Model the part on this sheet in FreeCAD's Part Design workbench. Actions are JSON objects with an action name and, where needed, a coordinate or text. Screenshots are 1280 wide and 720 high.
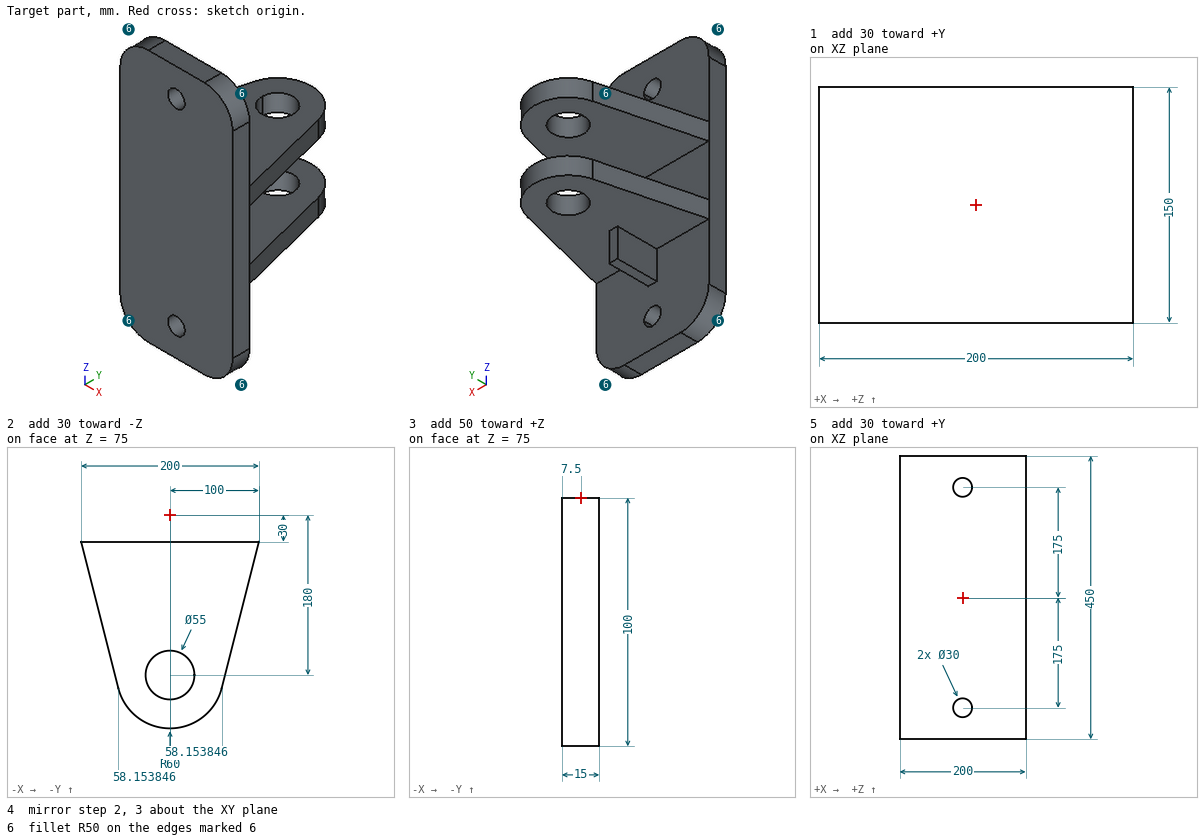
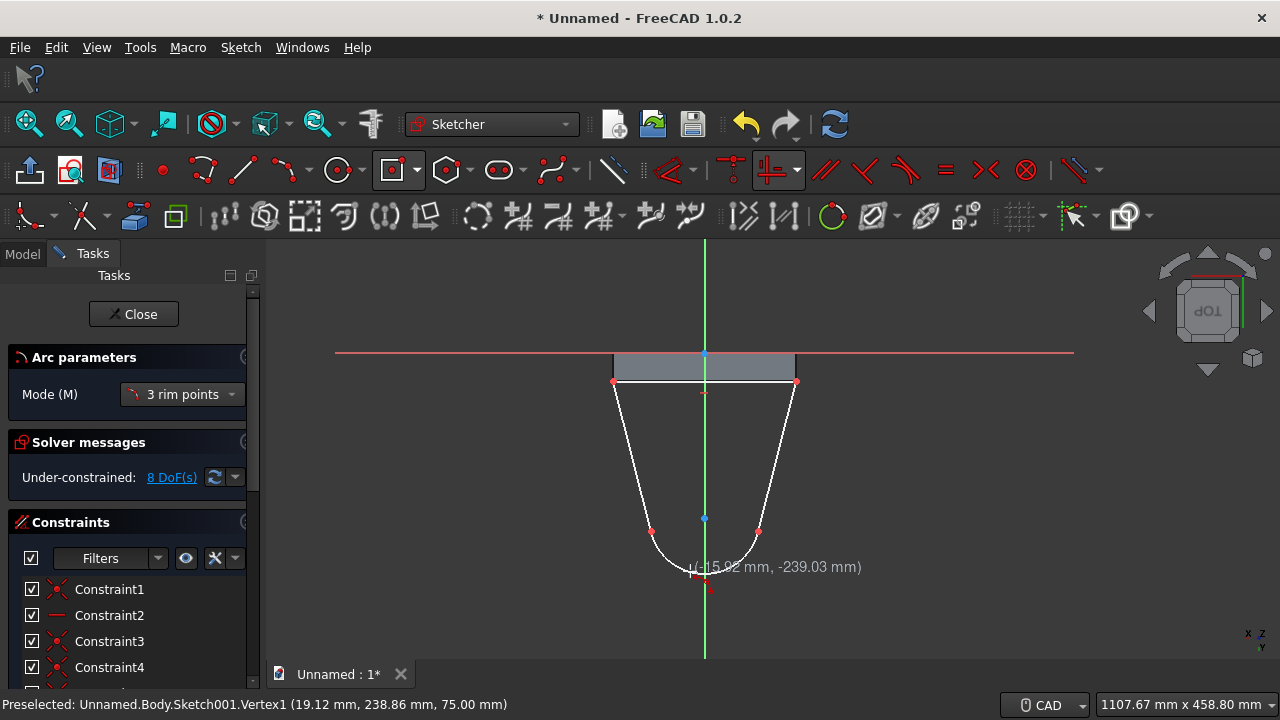
{"action": "key", "text": "g c"}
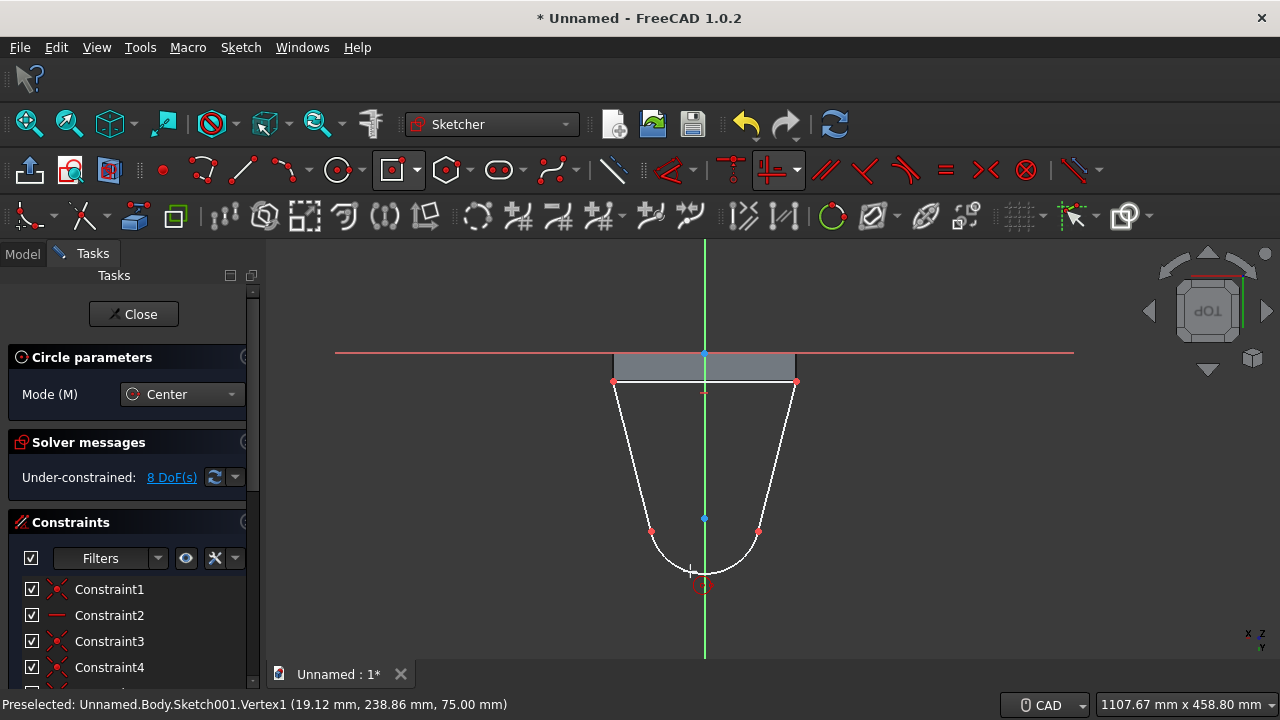
{"action": "left_click", "coordinate": [705, 518]}
{"action": "mouse_move", "coordinate": [722, 500]}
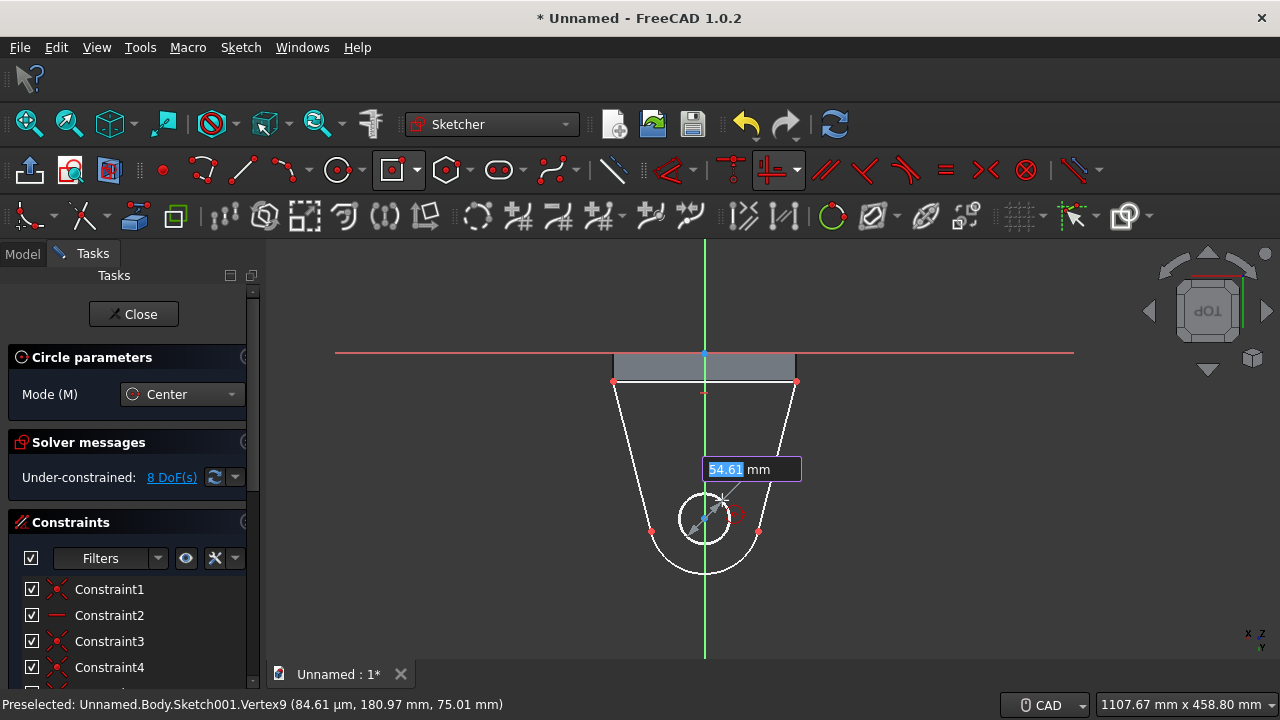
{"action": "type", "text": "55"}
{"action": "key", "text": "Return"}
{"action": "key", "text": "Escape"}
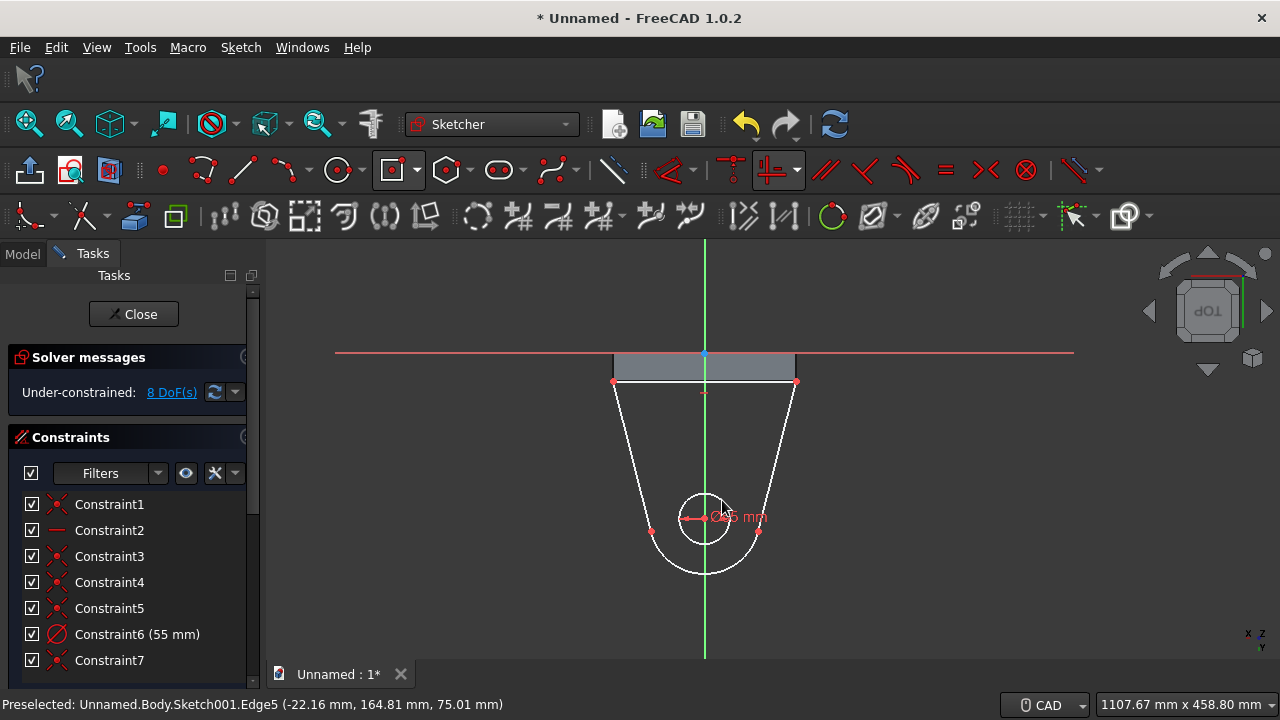
{"action": "left_click", "coordinate": [705, 519]}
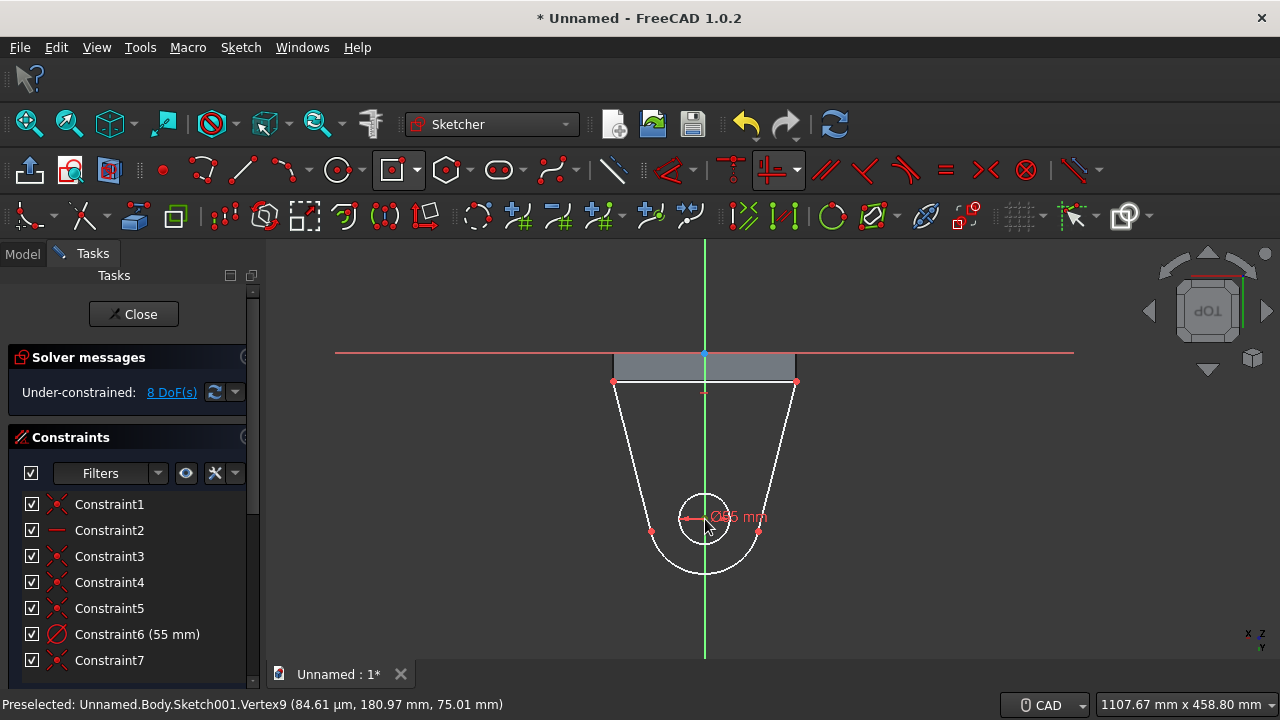
{"action": "left_click", "coordinate": [705, 605]}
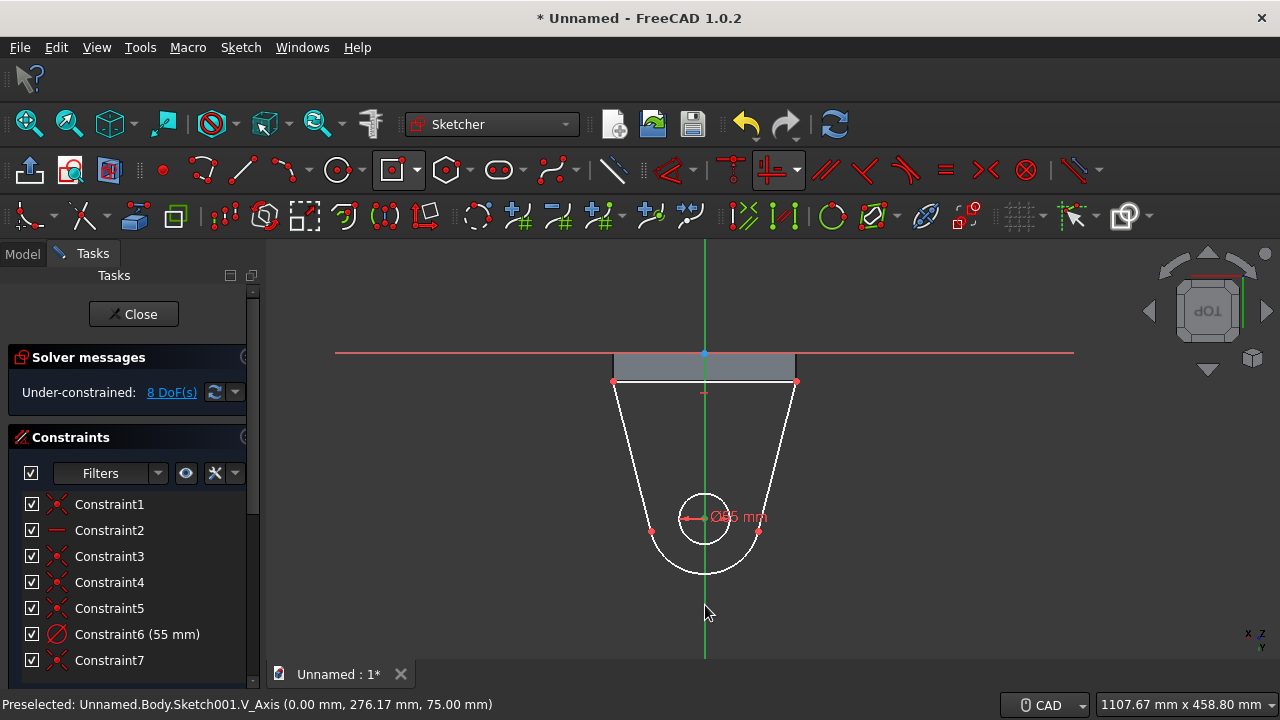
{"action": "left_click", "coordinate": [732, 170]}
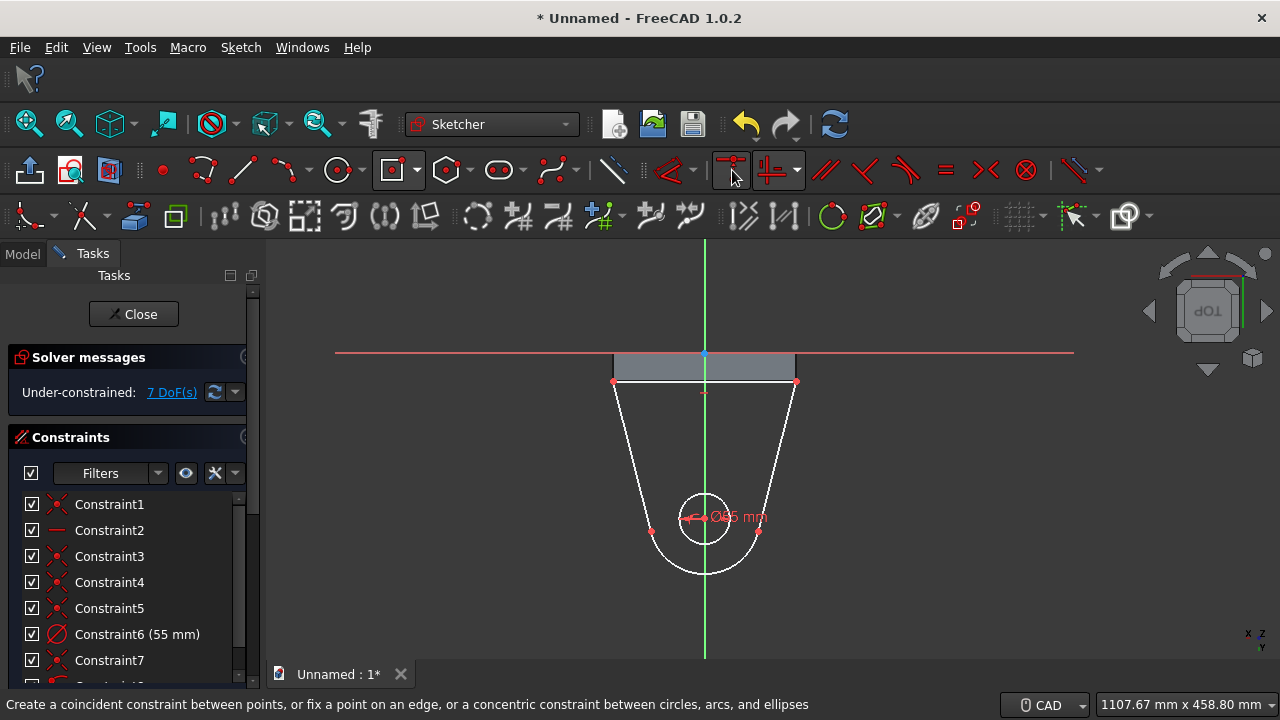
{"action": "key", "text": "d"}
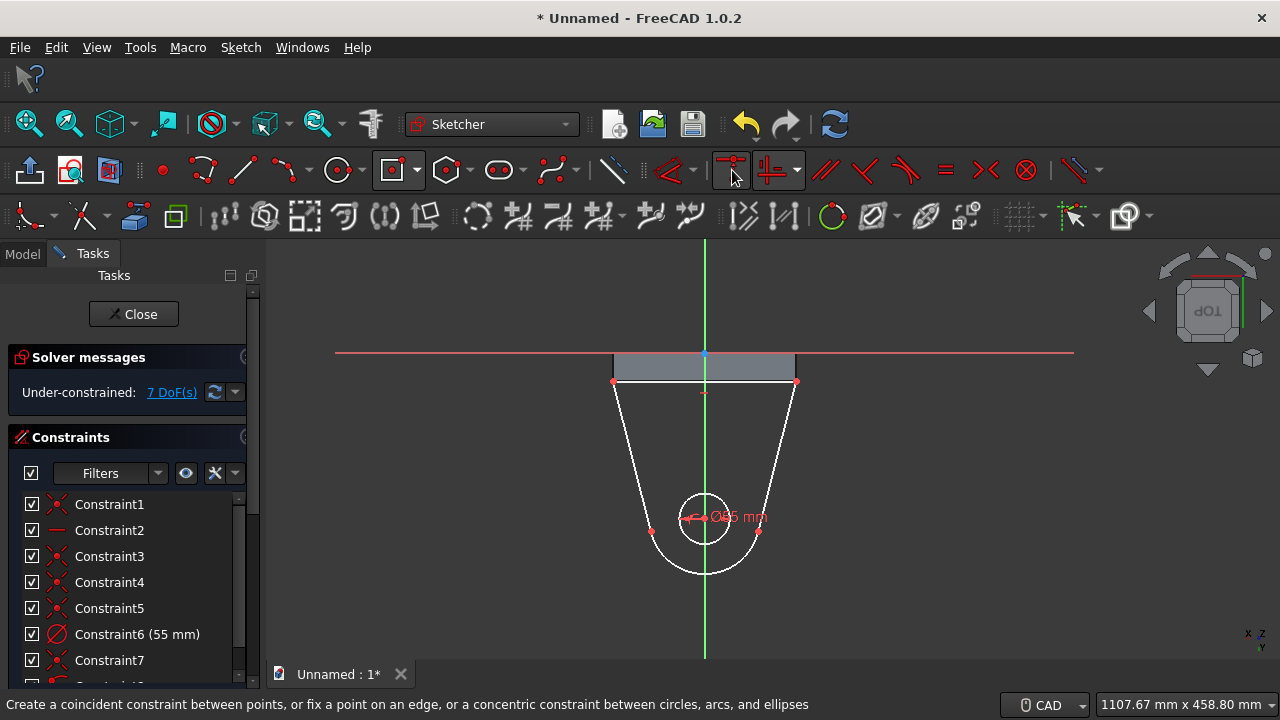
{"action": "left_click", "coordinate": [677, 566]}
{"action": "left_click", "coordinate": [661, 594]}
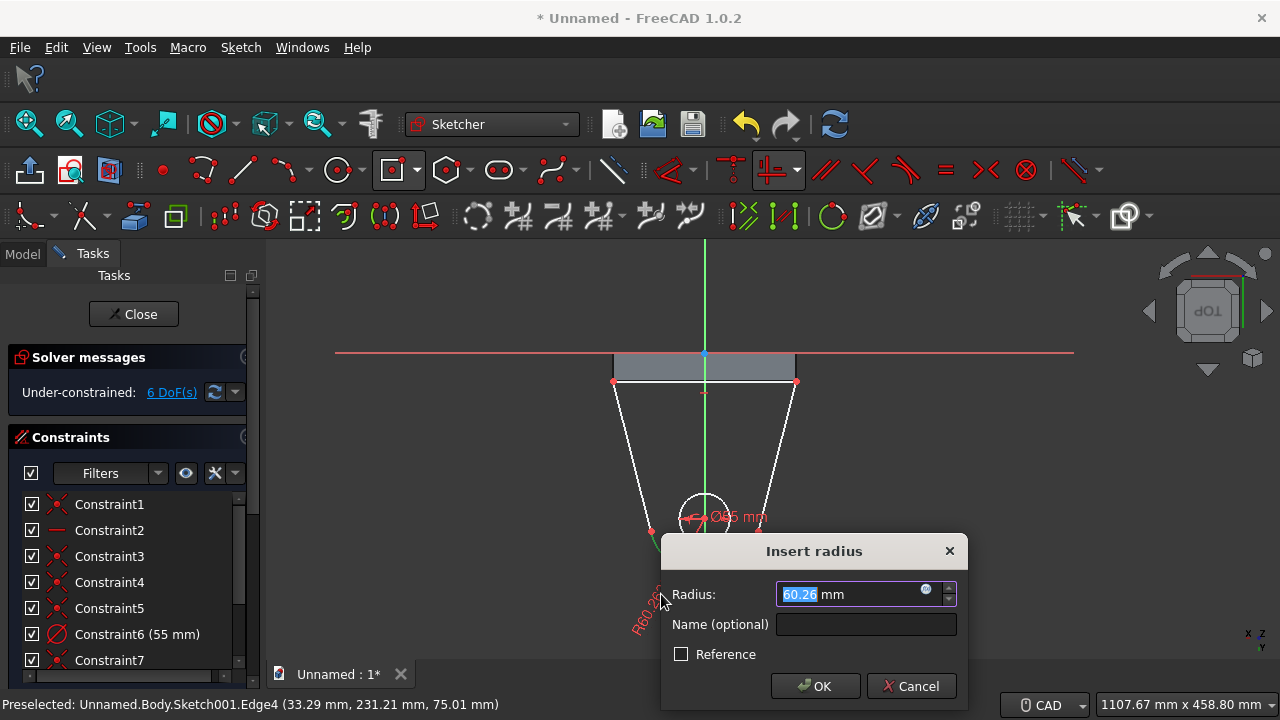
{"action": "type", "text": "60"}
{"action": "key", "text": "Return"}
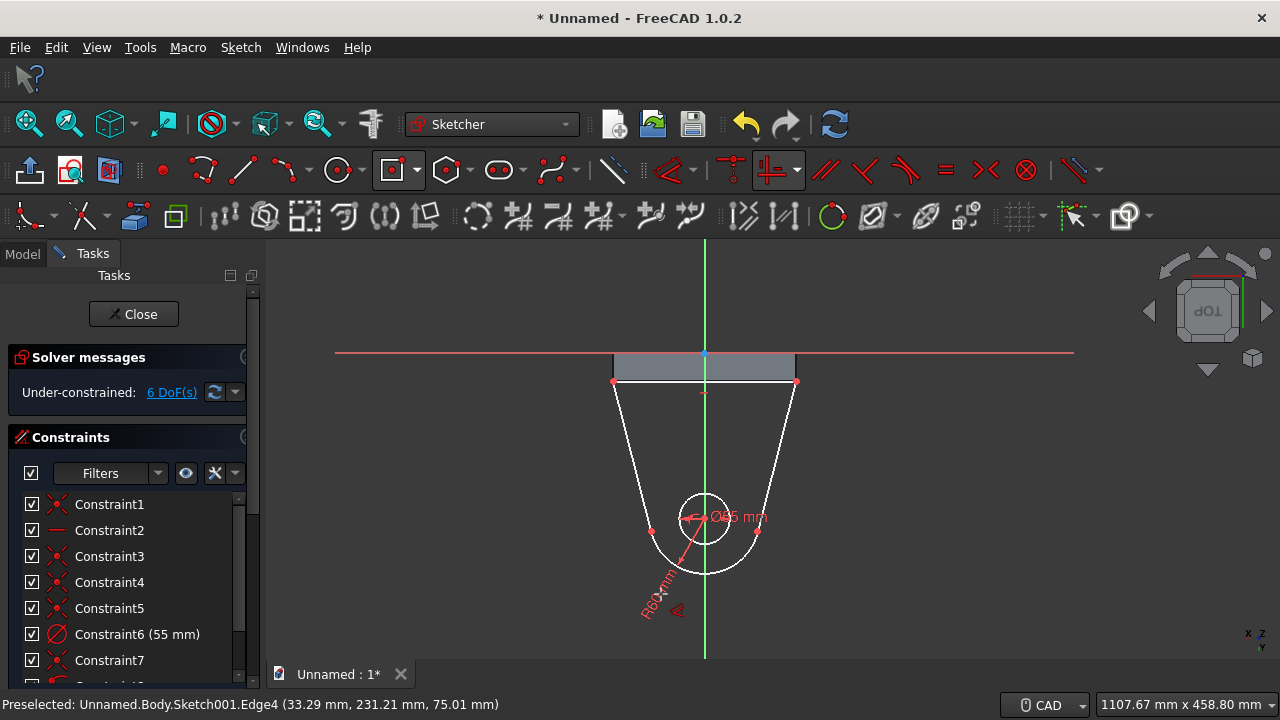
{"action": "left_click", "coordinate": [741, 382]}
{"action": "left_click", "coordinate": [662, 416]}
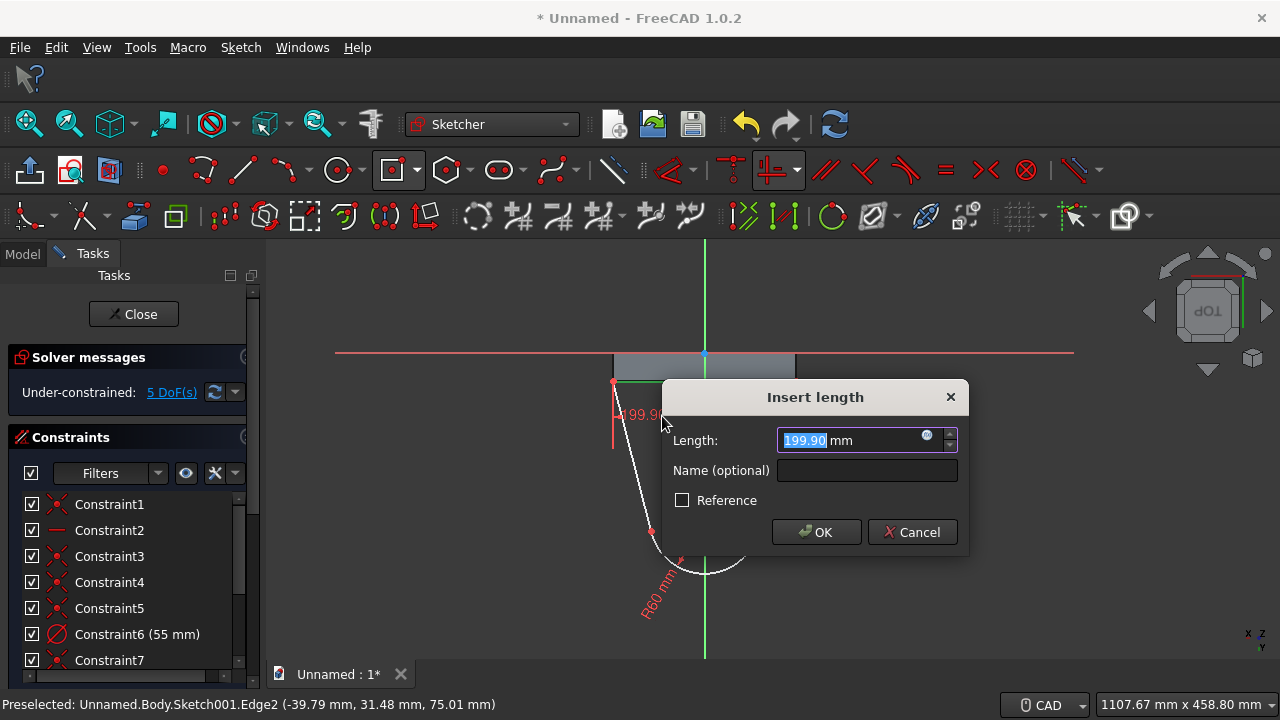
{"action": "type", "text": "200"}
{"action": "key", "text": "Return"}